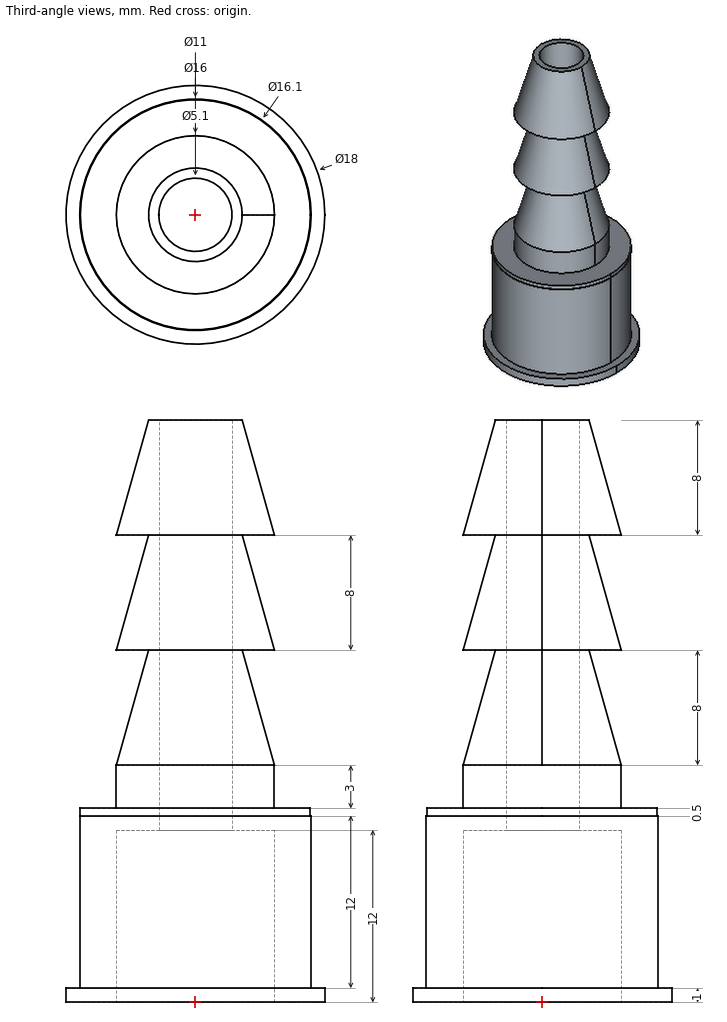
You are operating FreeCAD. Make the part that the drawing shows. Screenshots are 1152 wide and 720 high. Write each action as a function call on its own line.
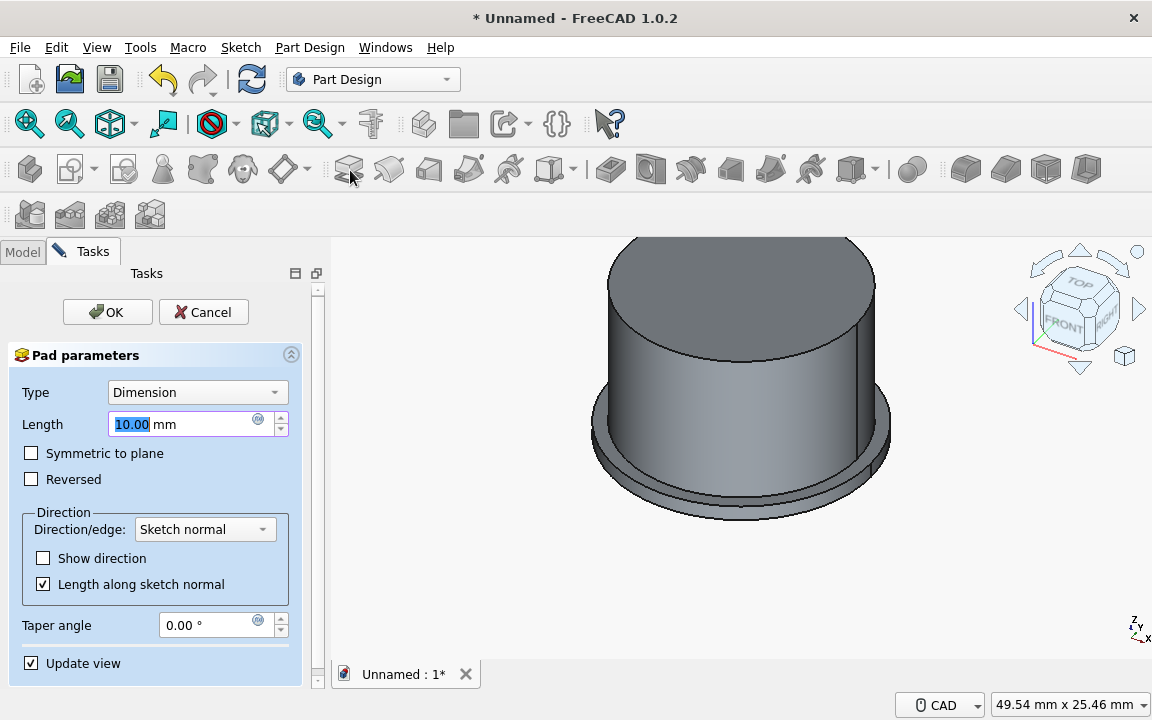
text(12)
key(Tab)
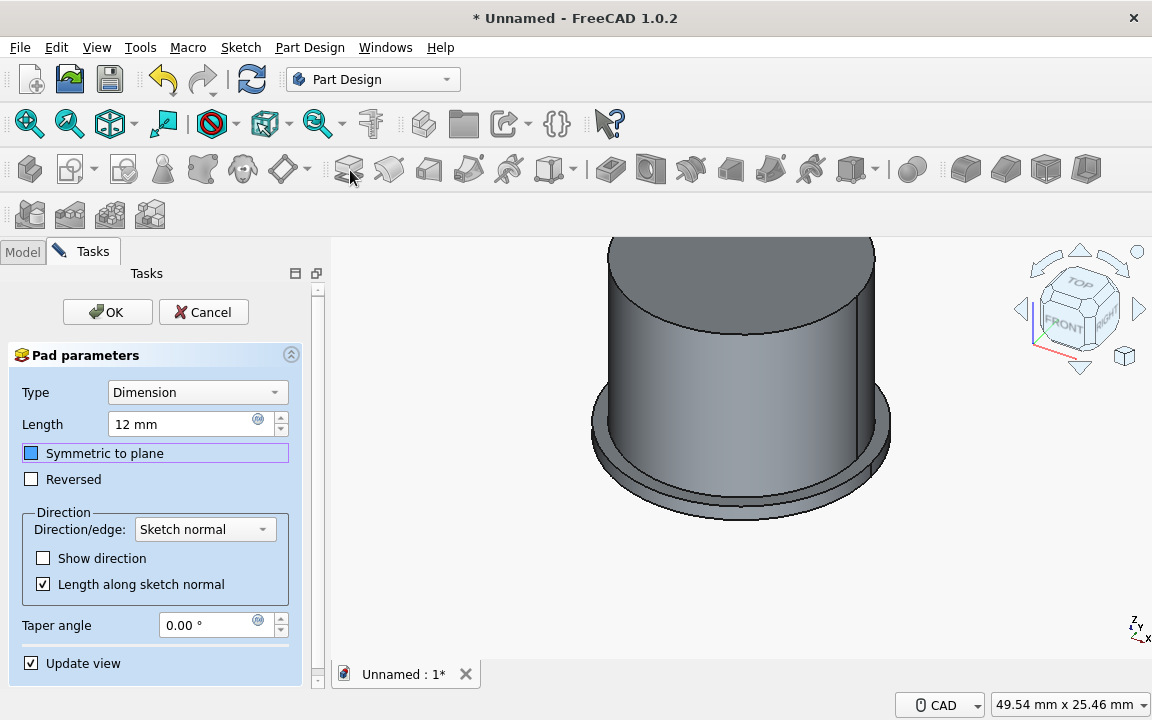
click(108, 312)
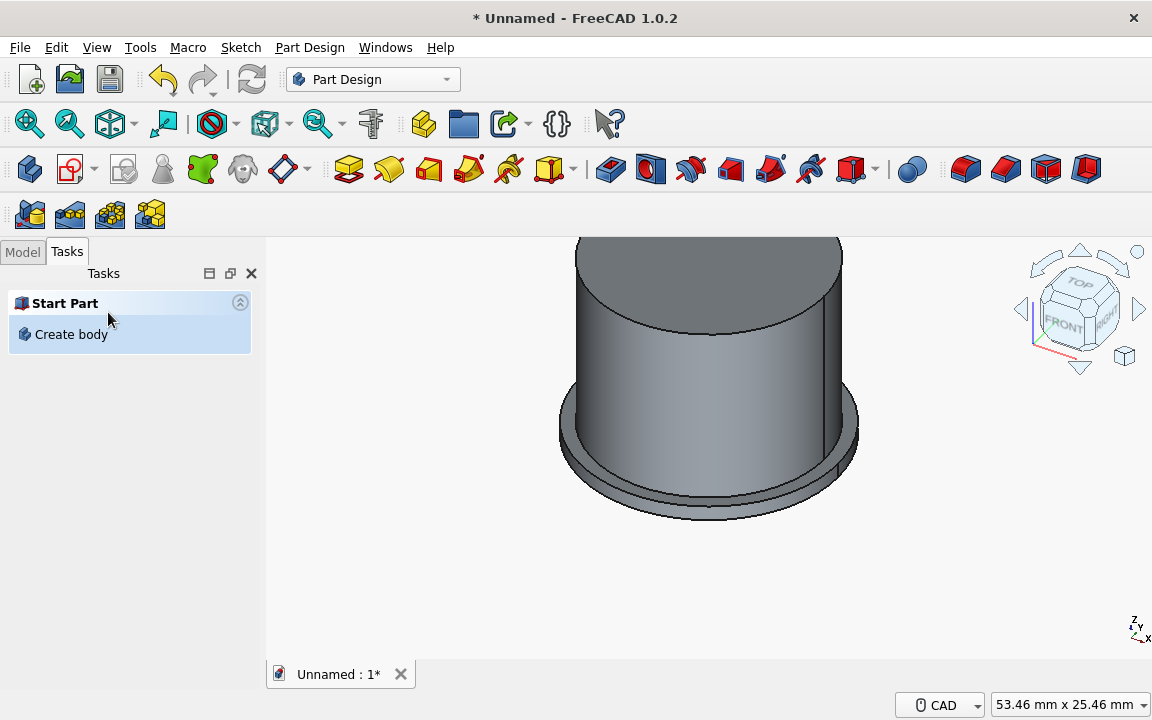
key(v)
key(f)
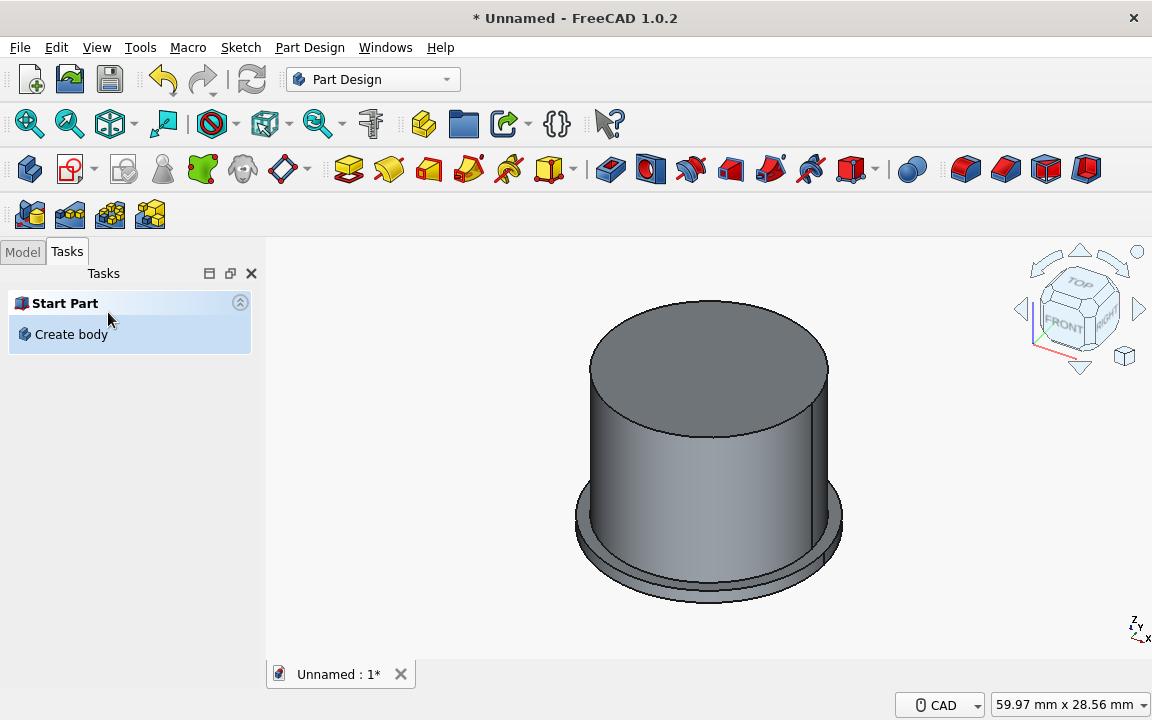
click(709, 368)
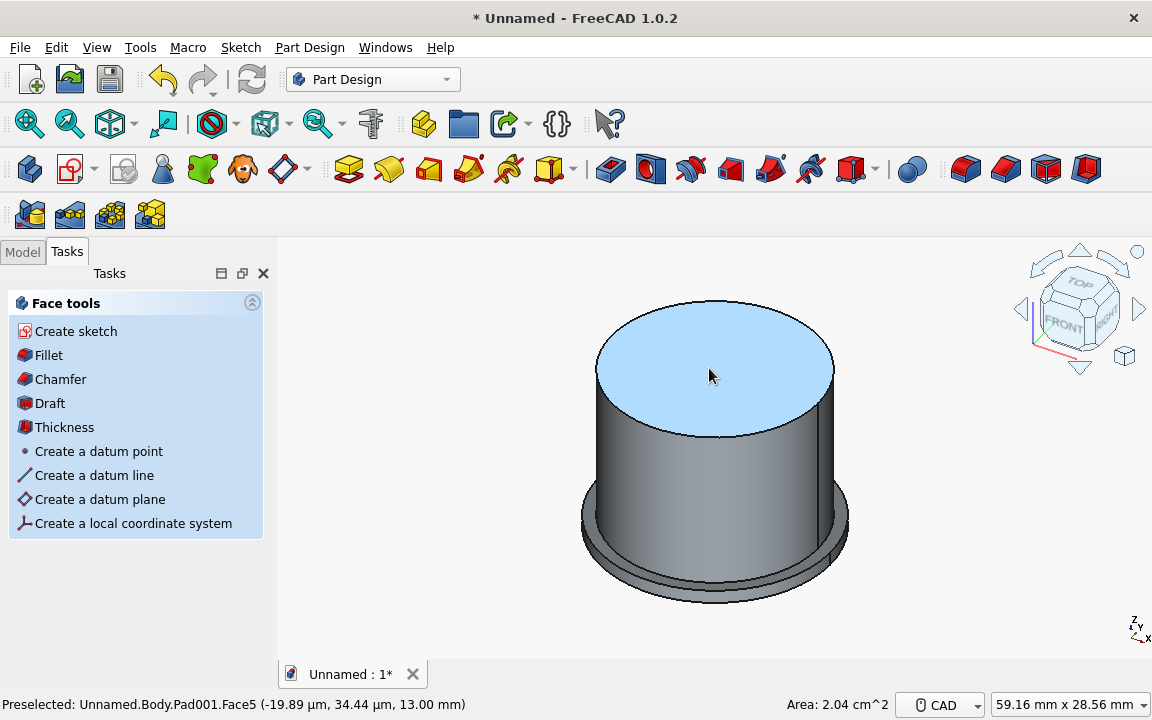
click(70, 170)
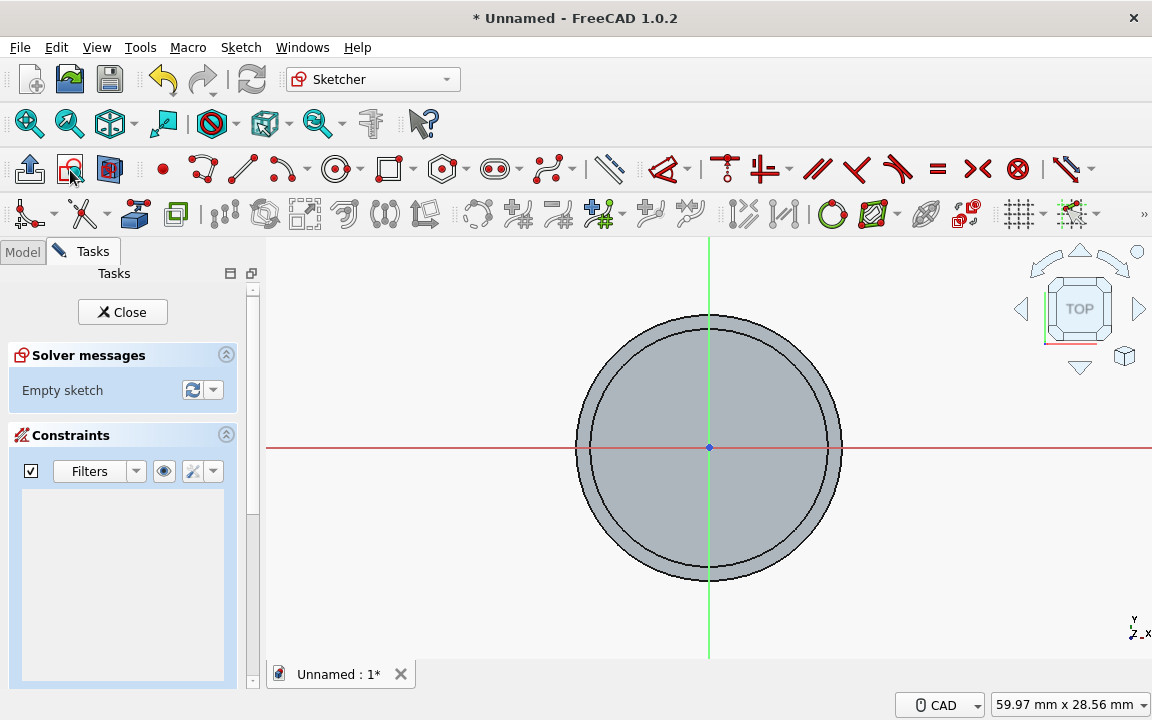
click(336, 170)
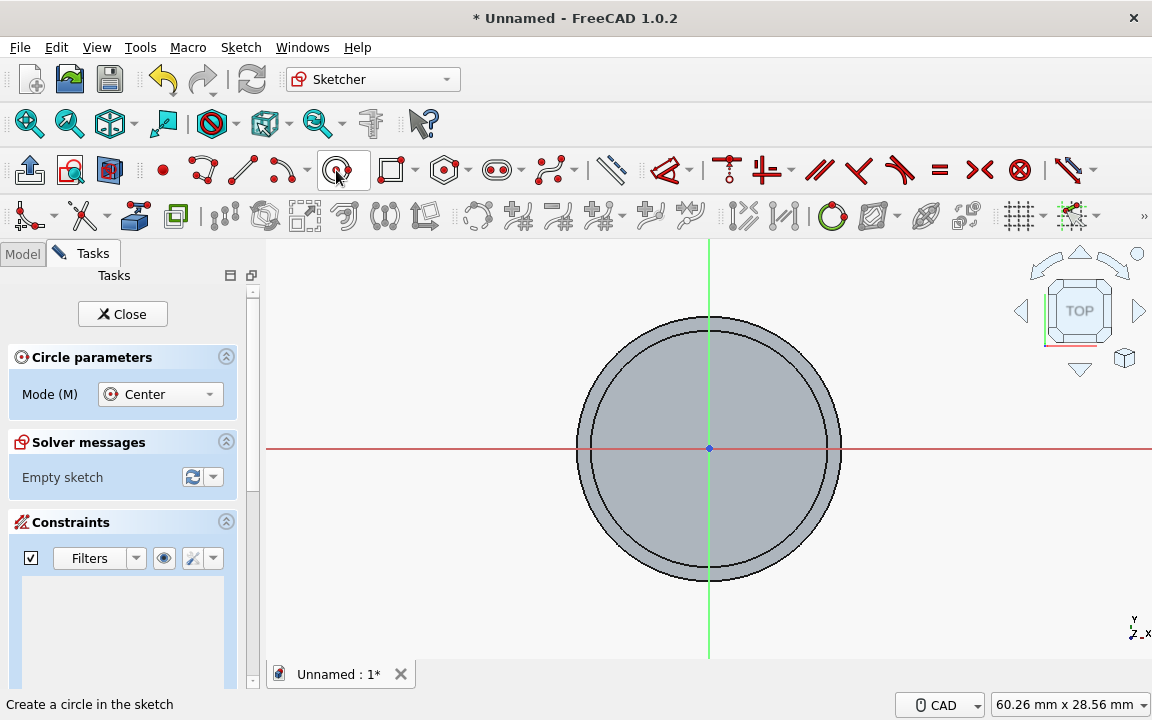
click(709, 449)
click(792, 366)
key(Escape)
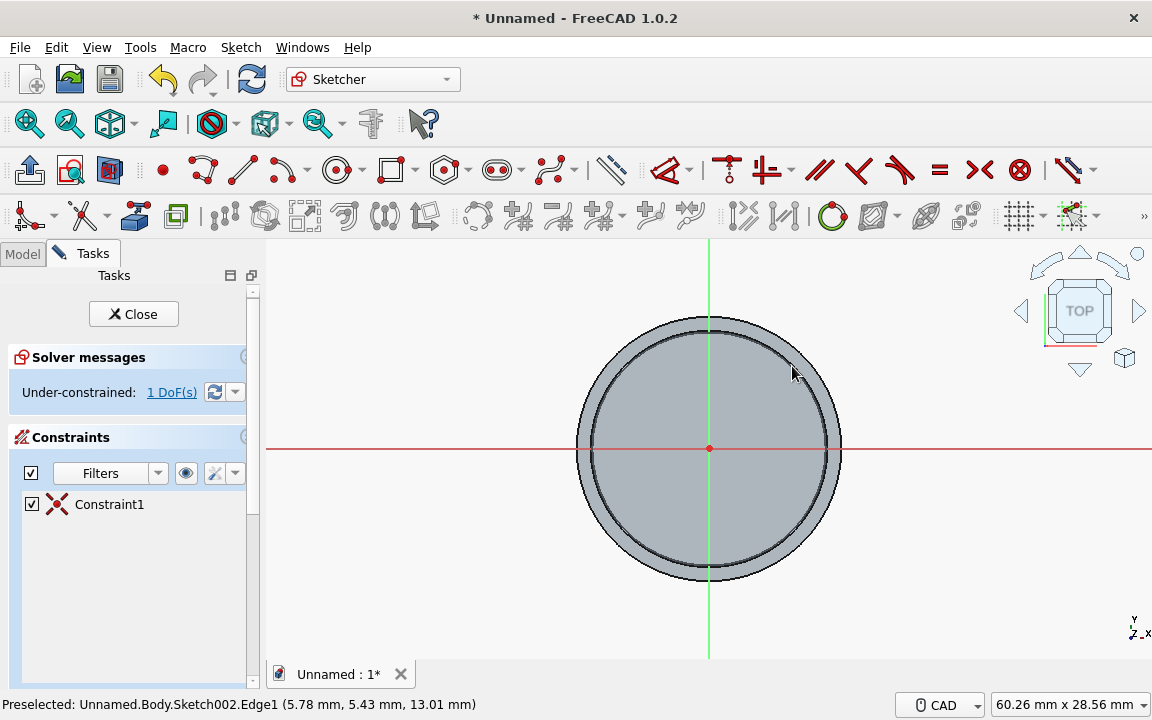
key(d)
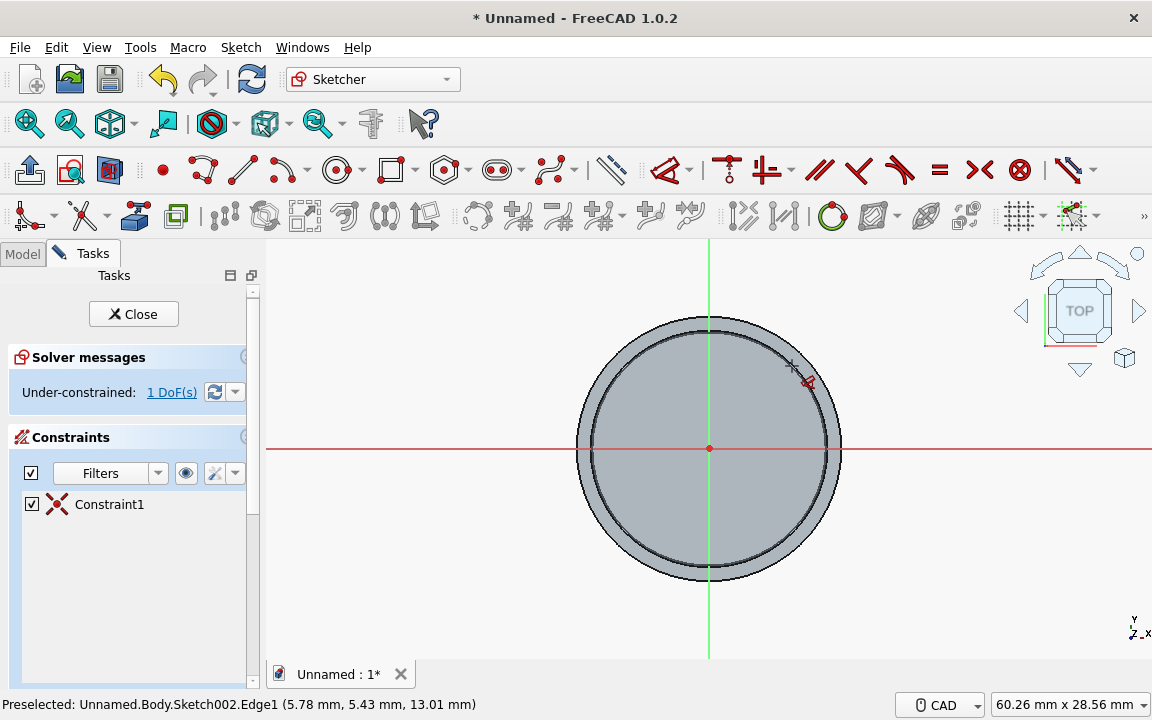
click(791, 366)
click(813, 343)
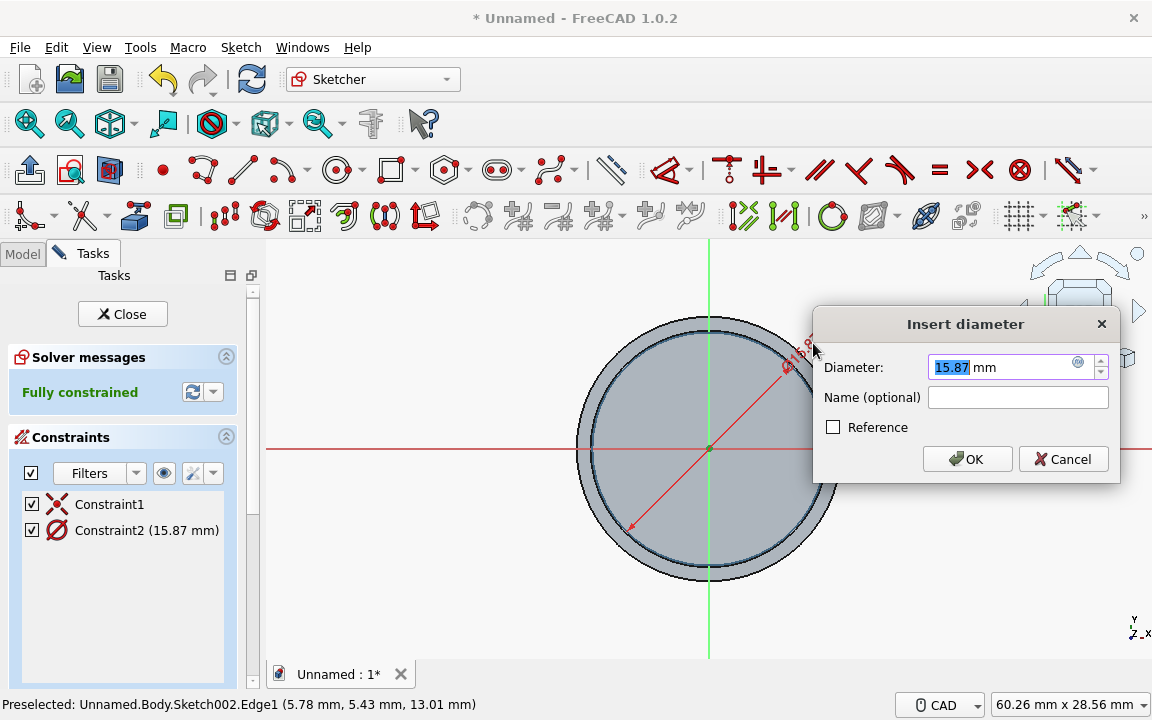
text(16)
key(Return)
key(Escape)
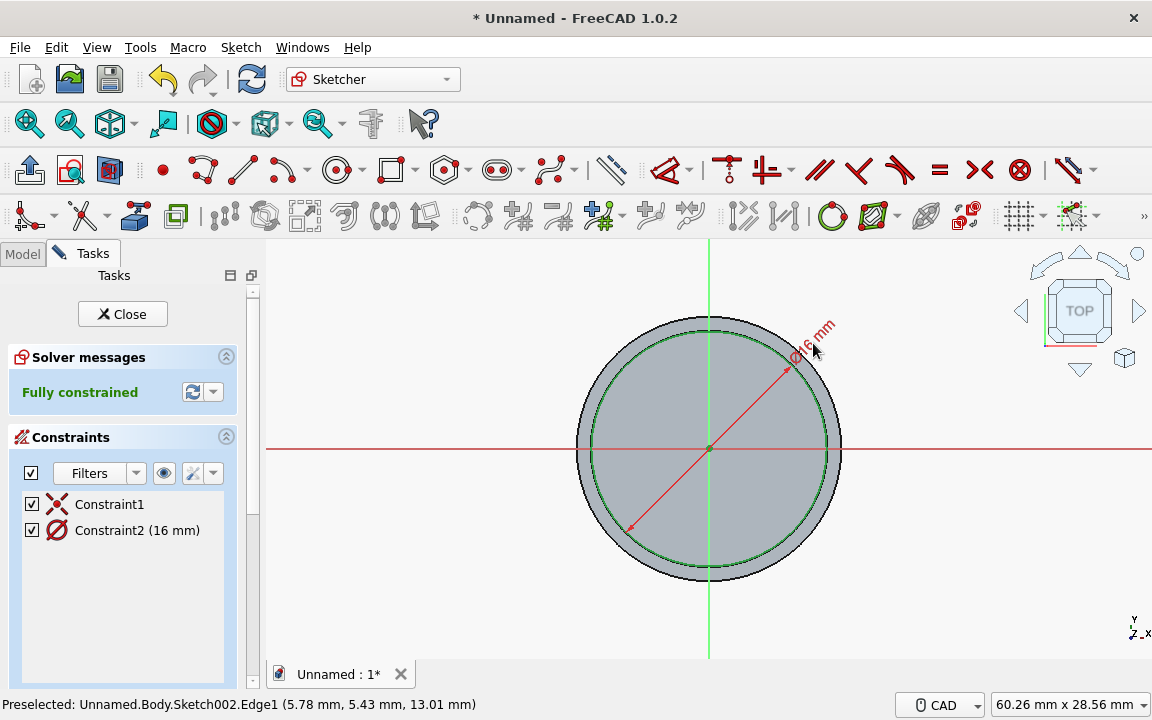
click(123, 314)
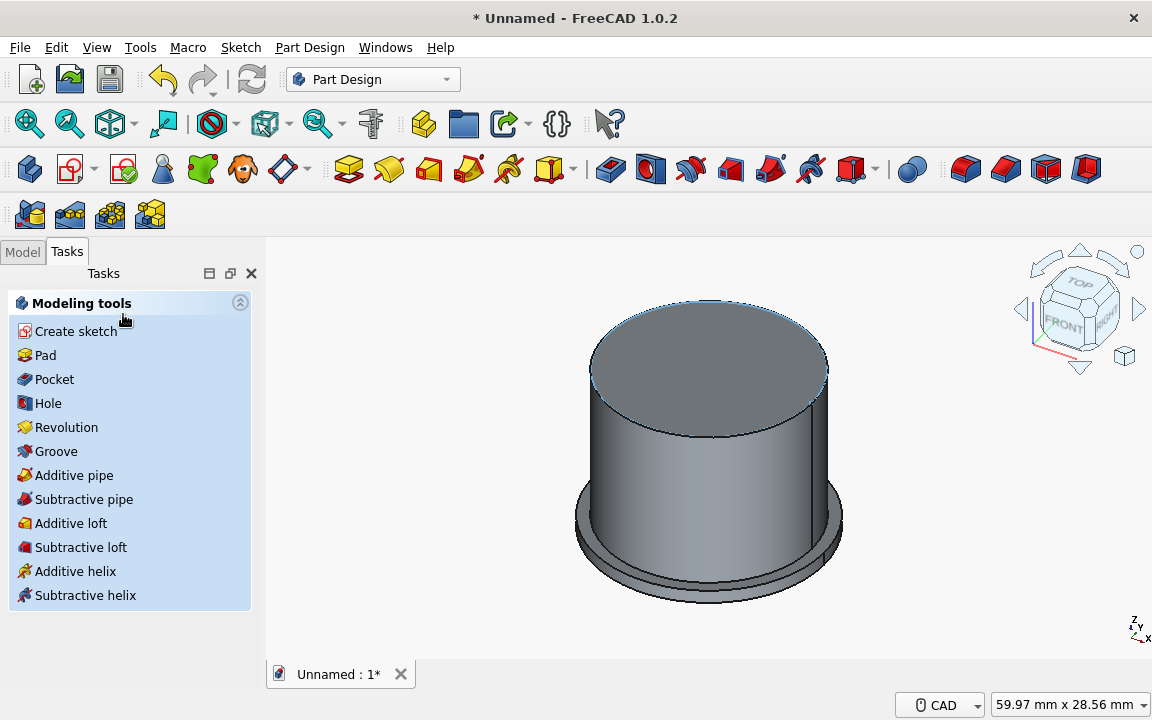
click(350, 170)